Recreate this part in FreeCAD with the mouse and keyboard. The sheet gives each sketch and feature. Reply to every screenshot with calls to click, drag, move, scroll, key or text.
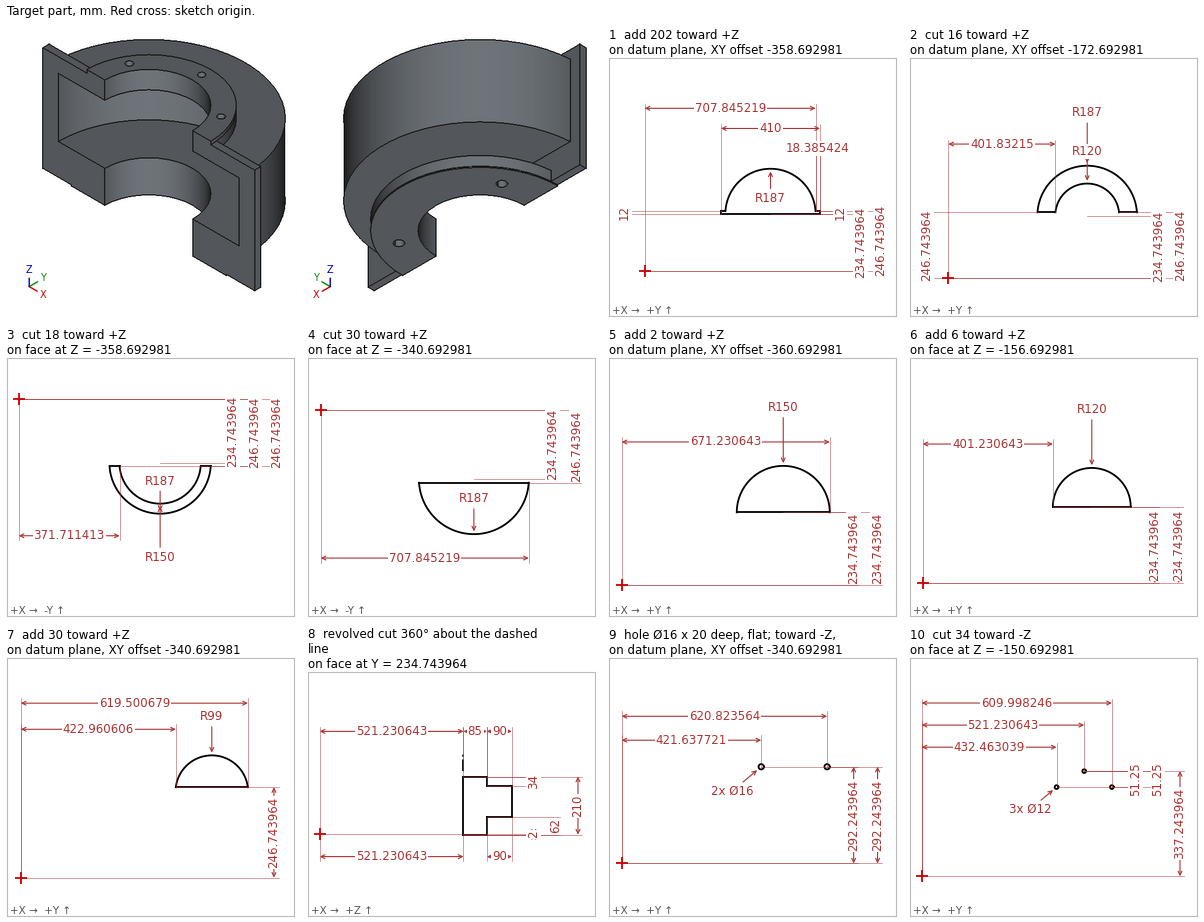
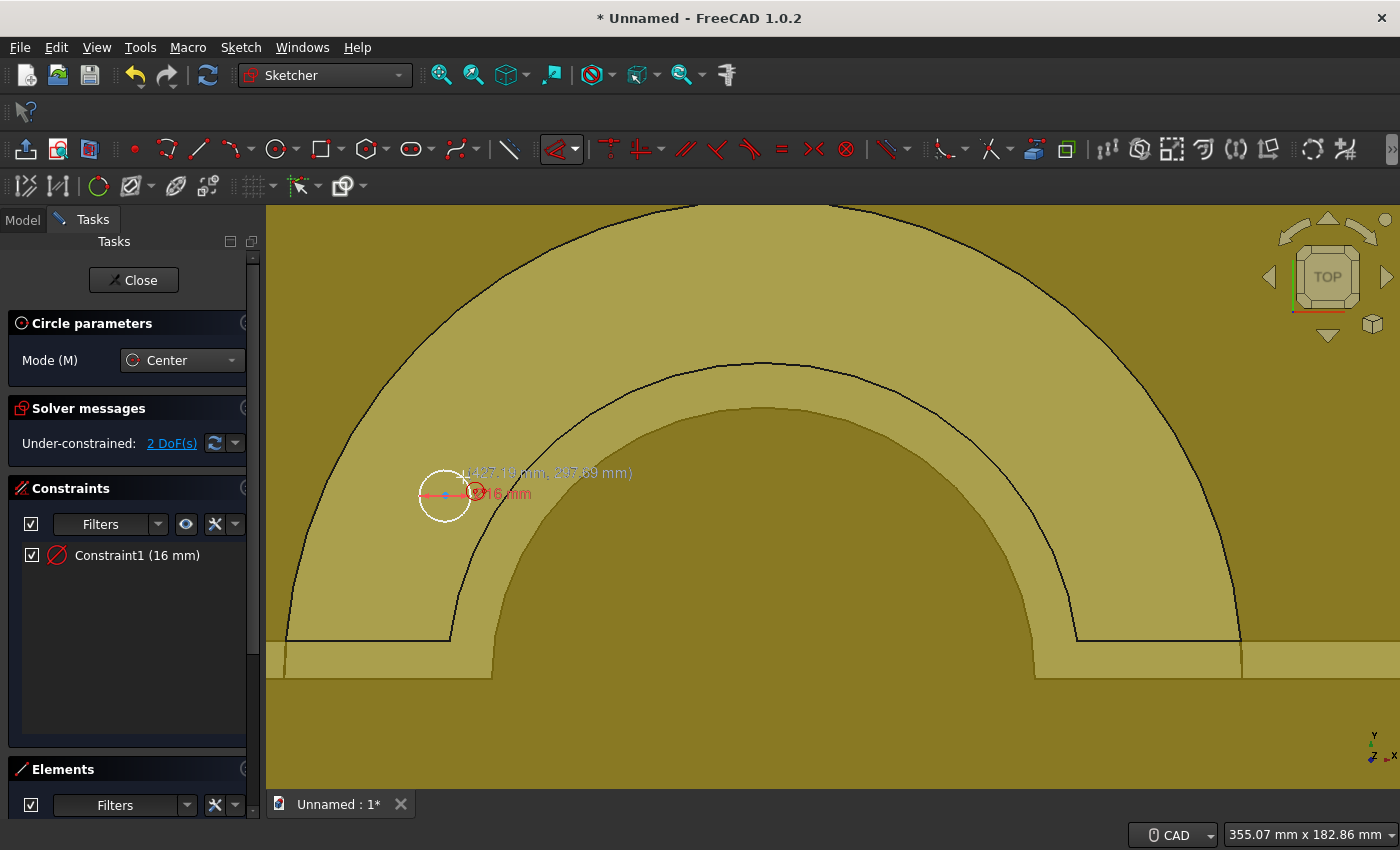
click(1081, 495)
move(1099, 477)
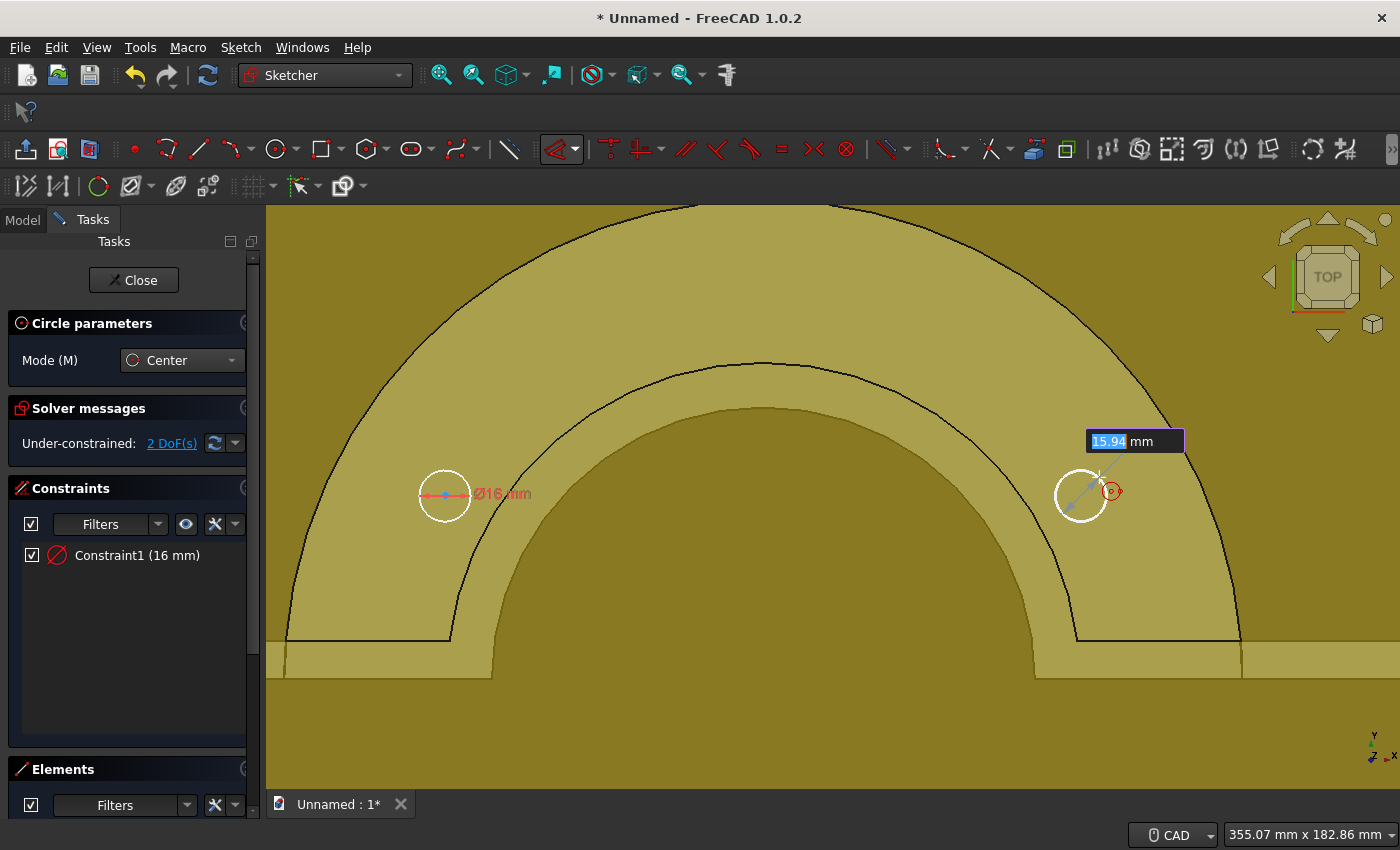
text(16)
key(Return)
key(Escape)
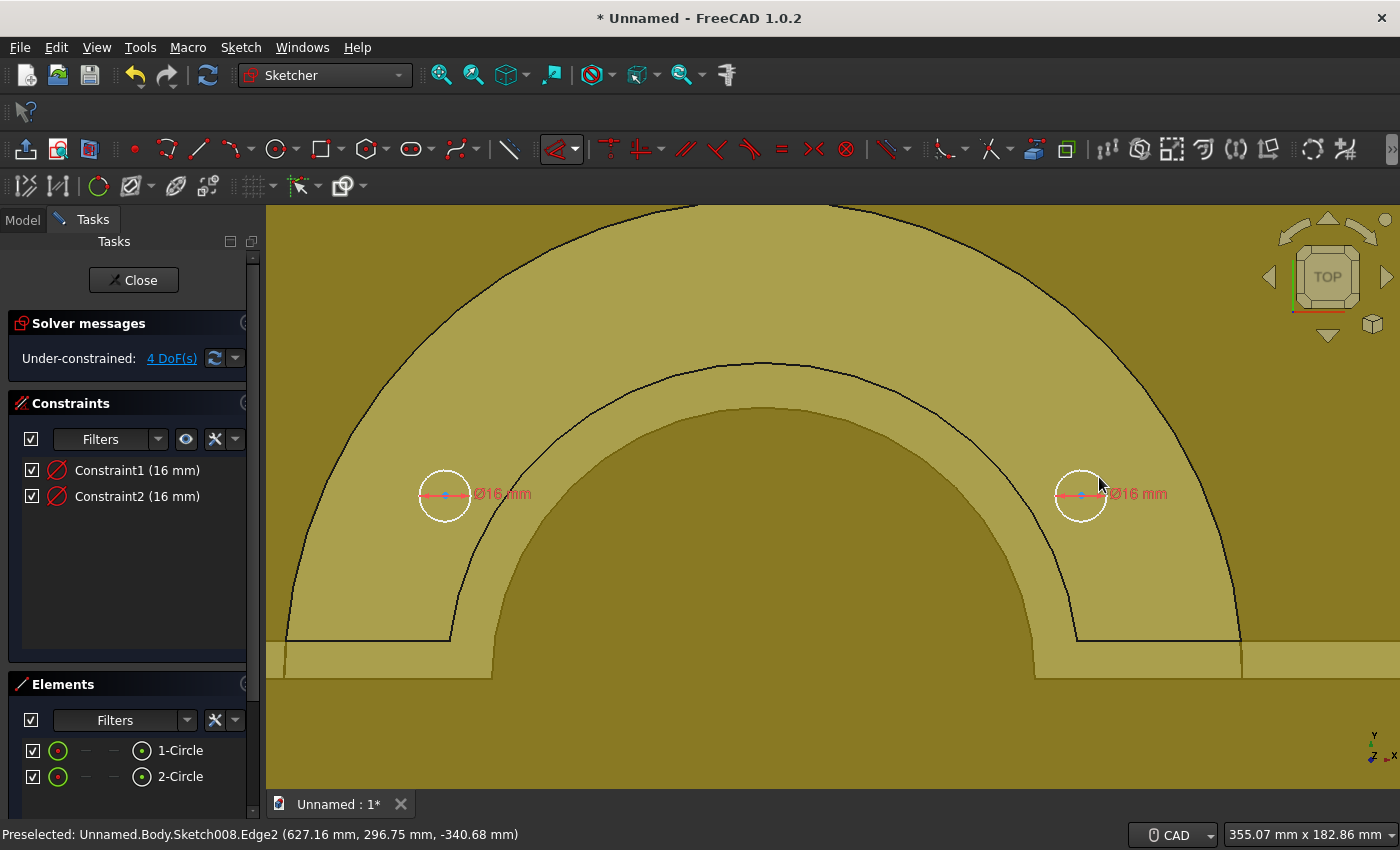
click(556, 150)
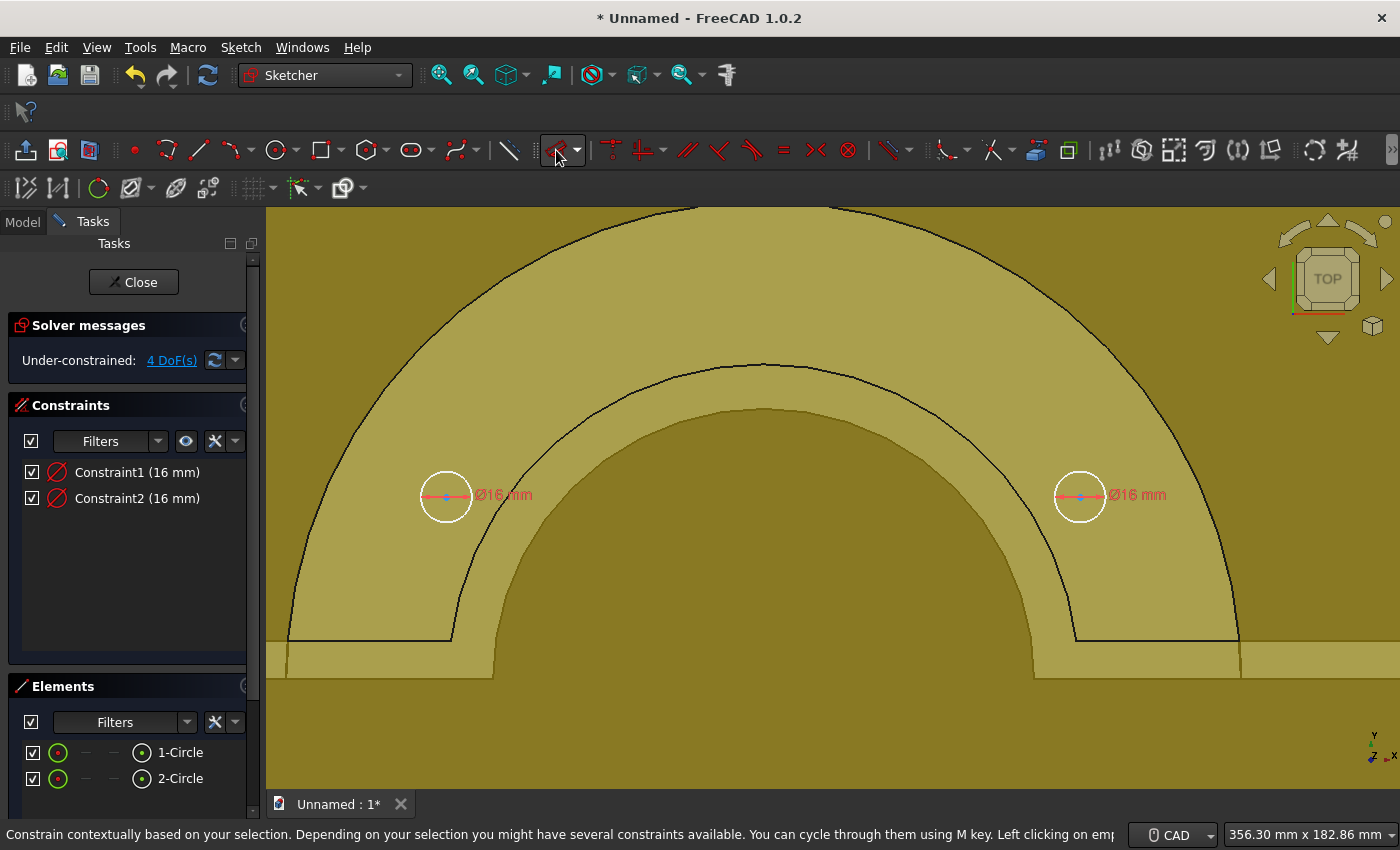
click(446, 497)
click(370, 463)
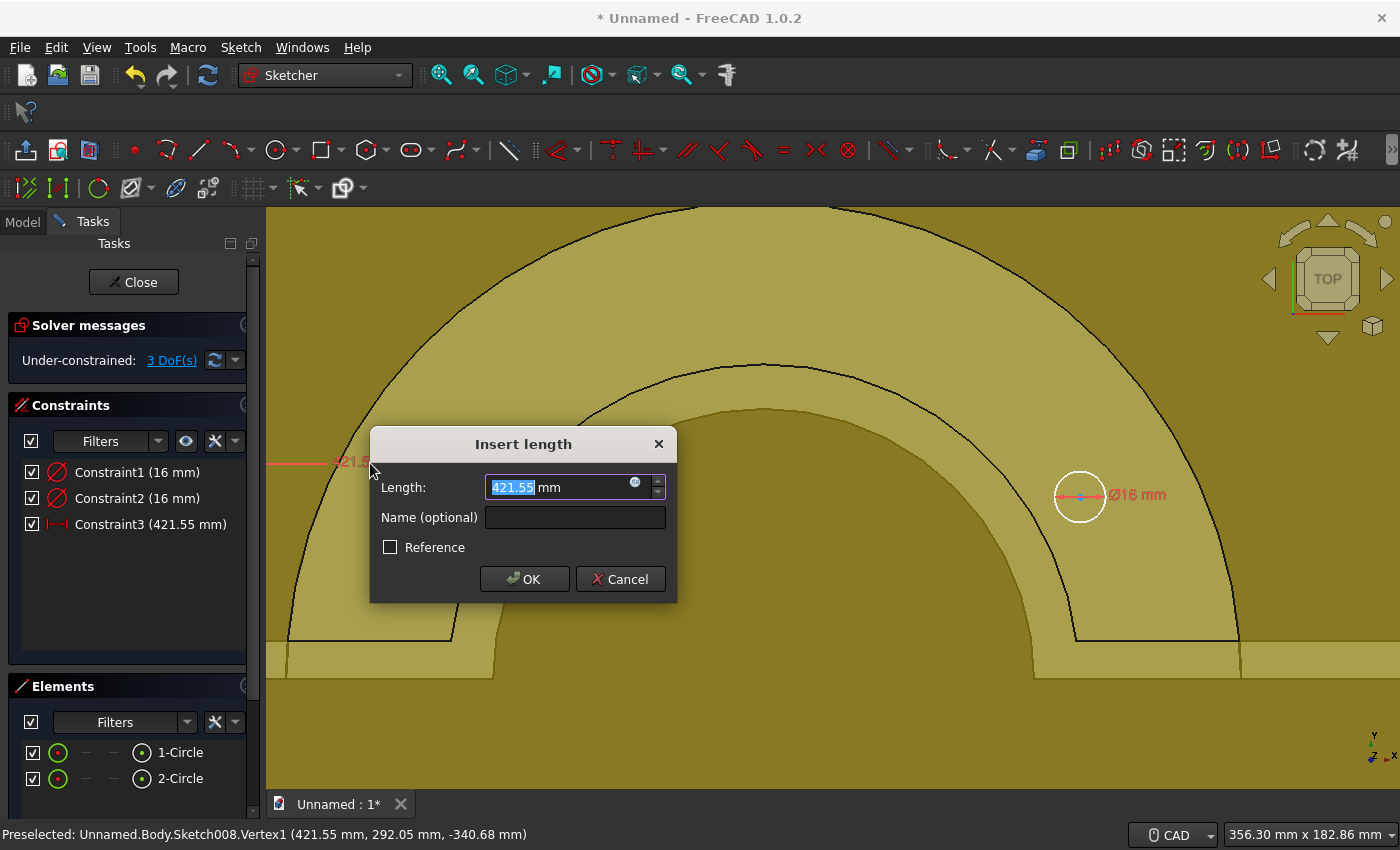
text(421.637721)
key(Return)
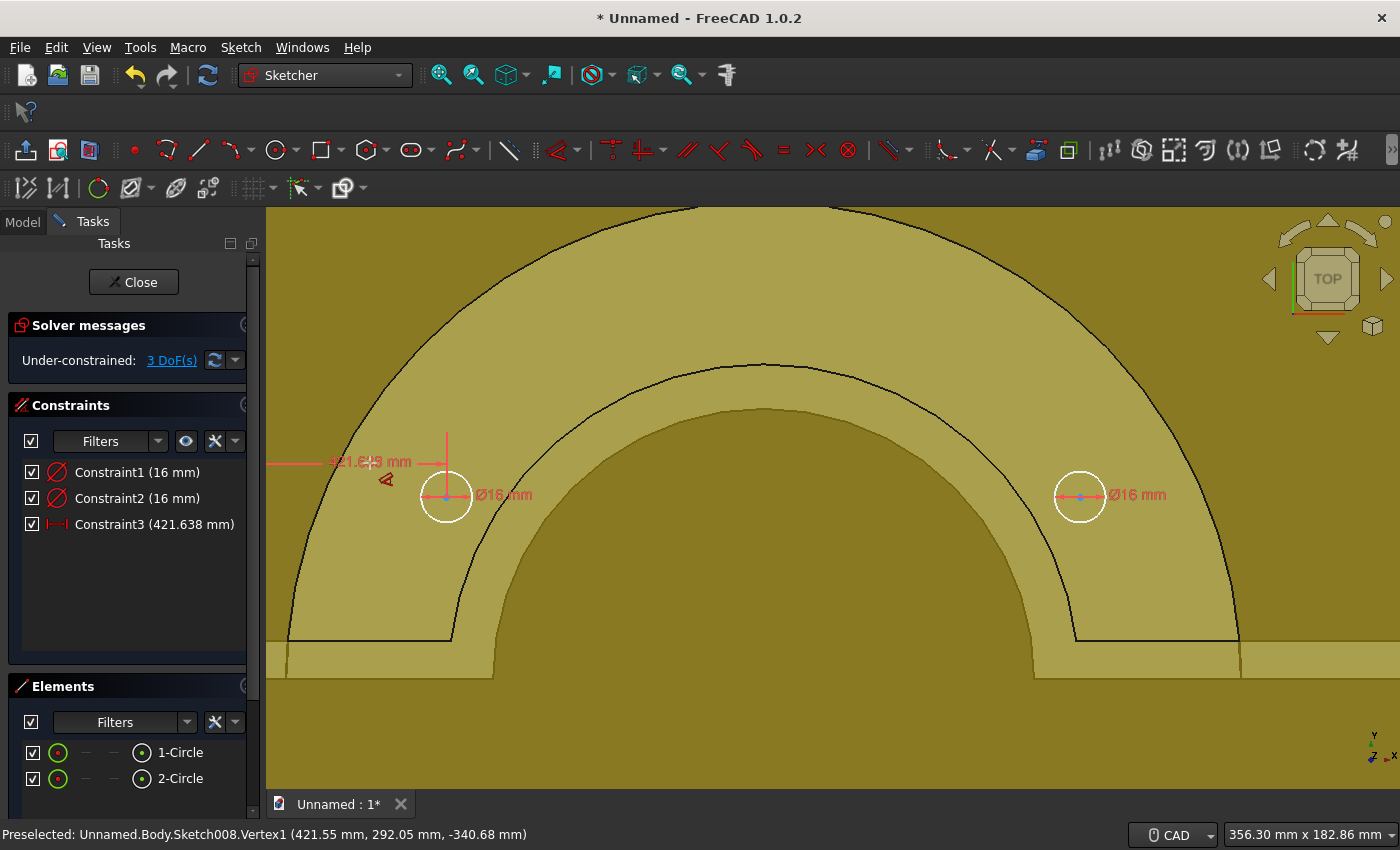
click(447, 497)
click(481, 629)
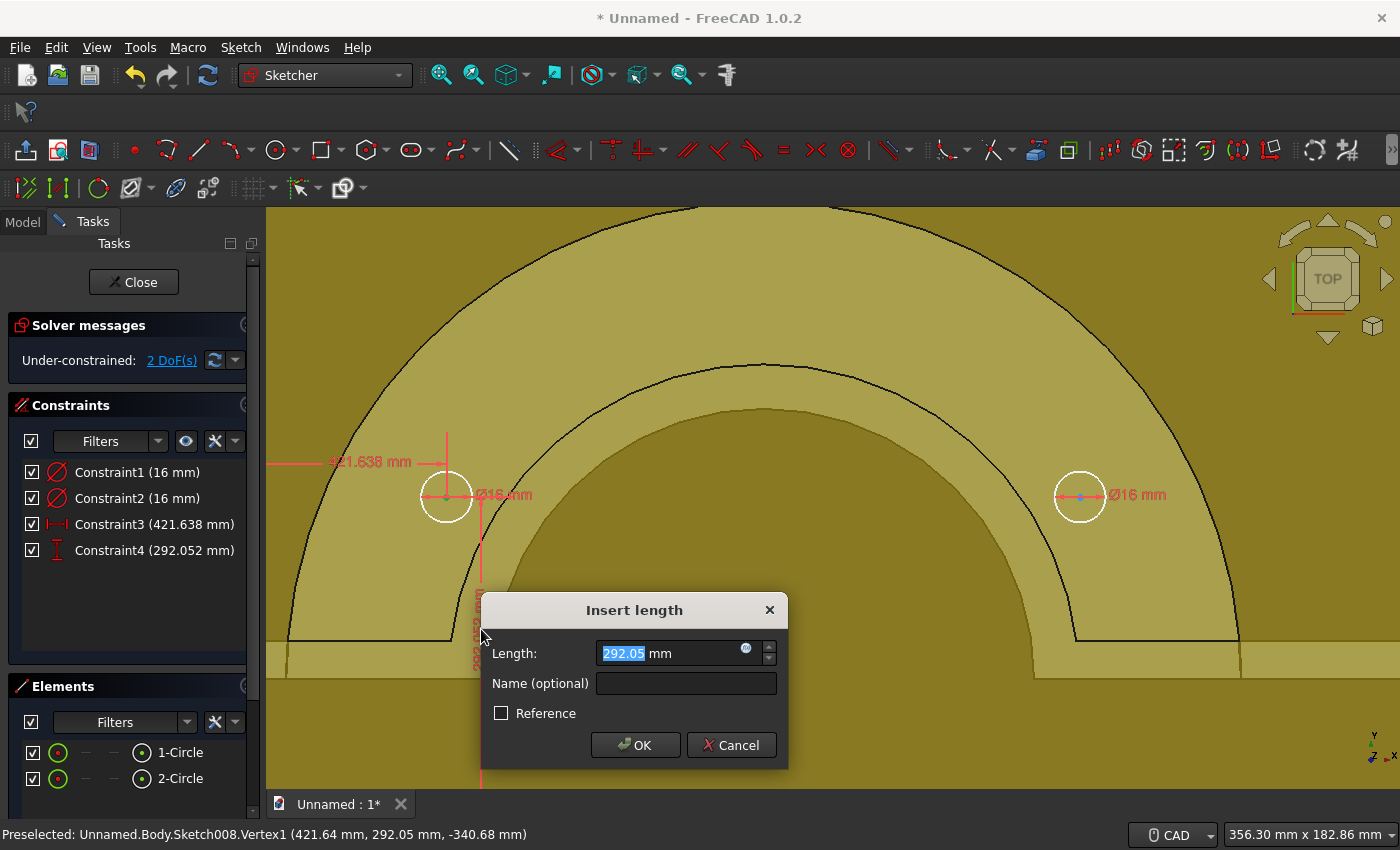
text(292.243964)
key(Return)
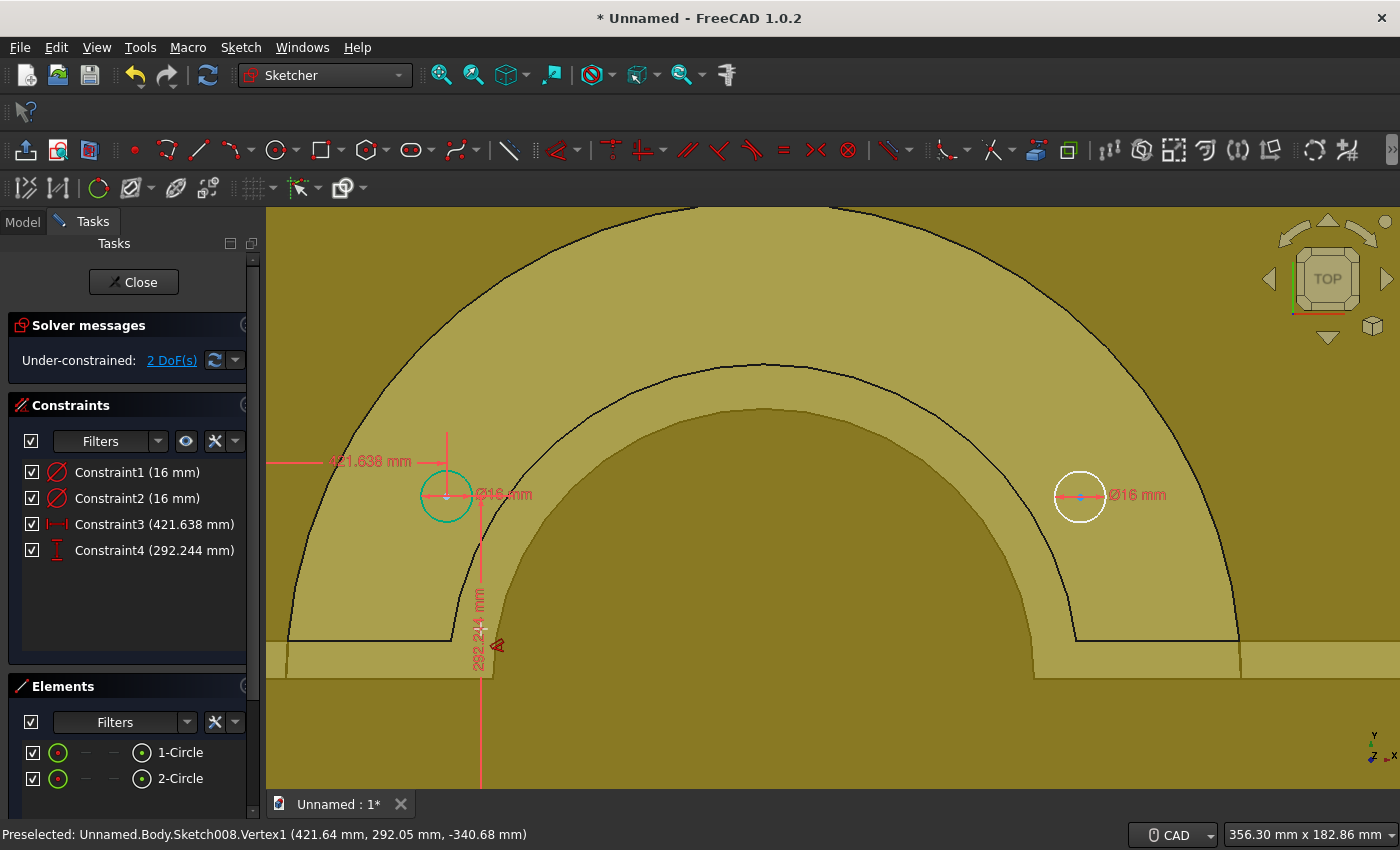
click(1080, 497)
click(687, 463)